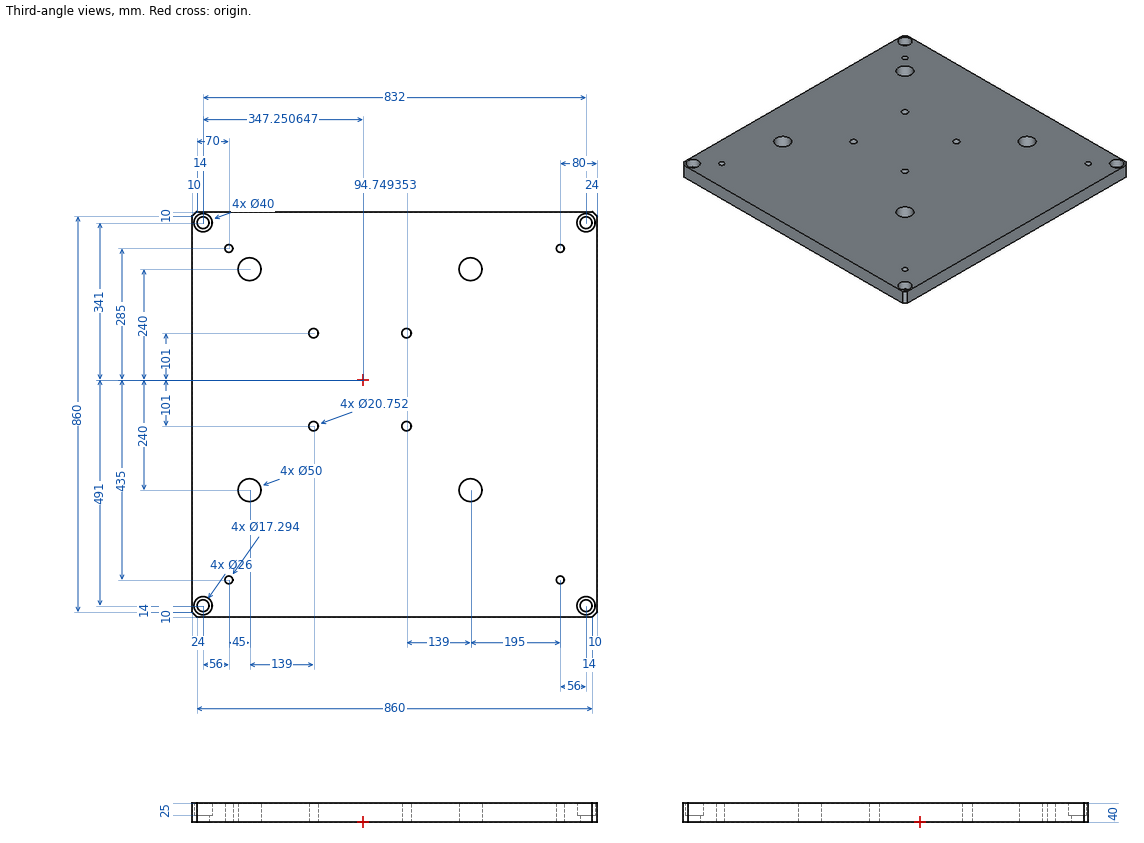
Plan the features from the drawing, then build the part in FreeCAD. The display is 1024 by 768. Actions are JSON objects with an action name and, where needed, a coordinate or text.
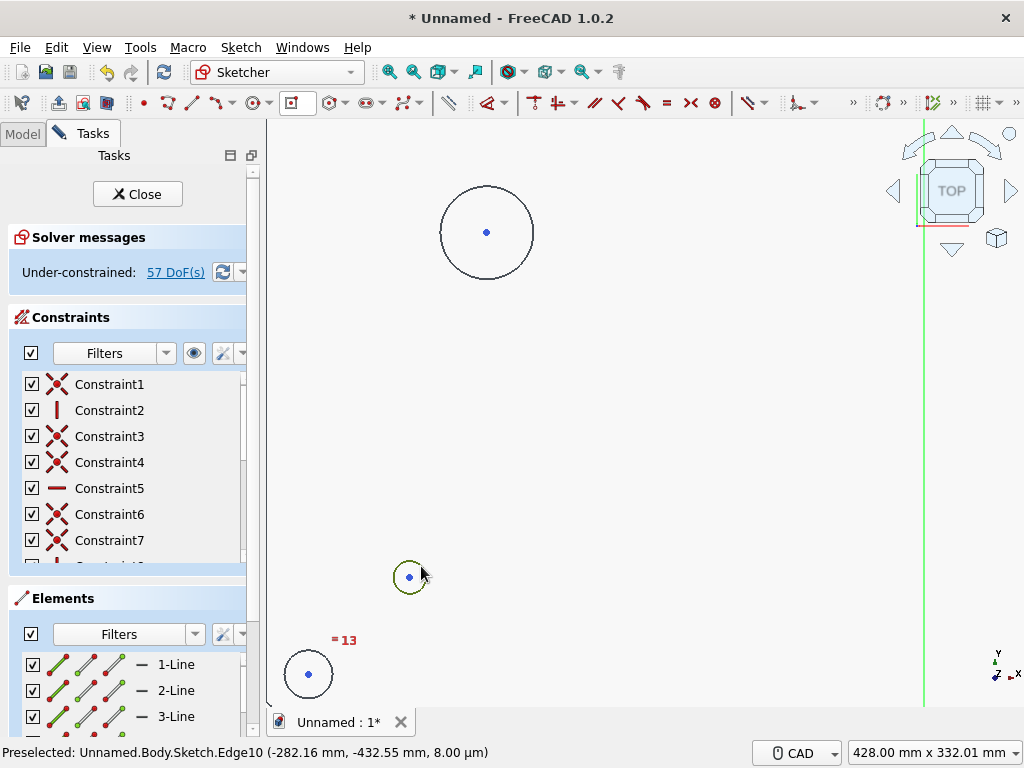
{"action": "scroll", "coordinate": [423, 569], "scroll_direction": "down", "scroll_amount": 7}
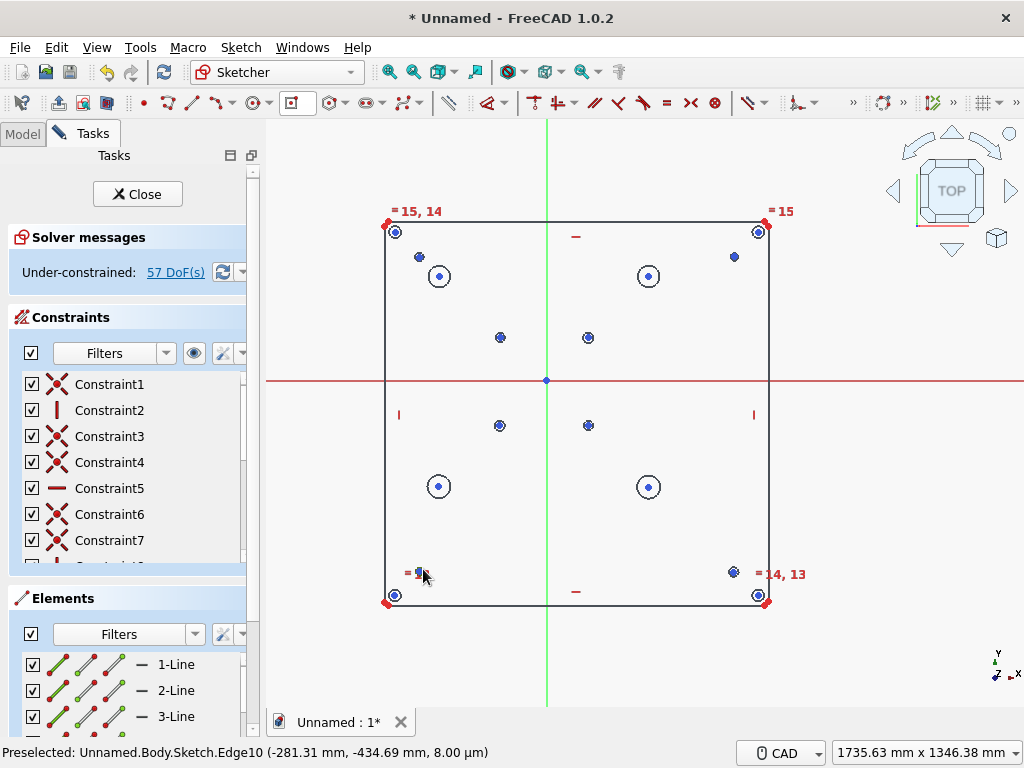
{"action": "scroll", "coordinate": [737, 569], "scroll_direction": "up", "scroll_amount": 6}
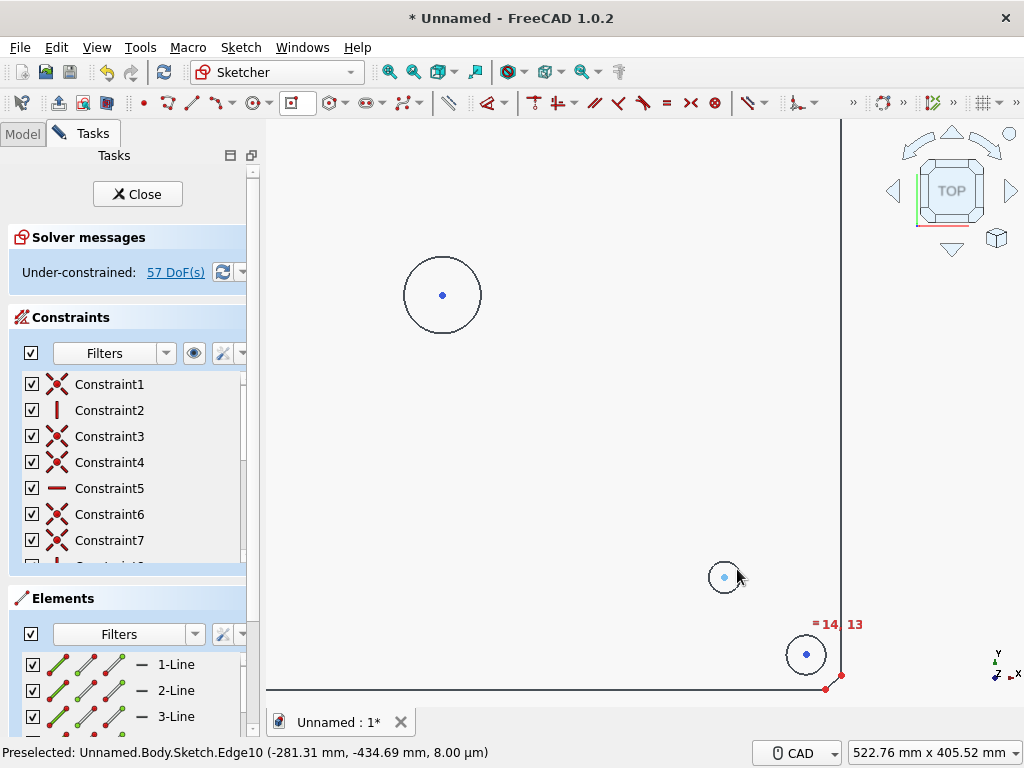
{"action": "left_click", "coordinate": [736, 566]}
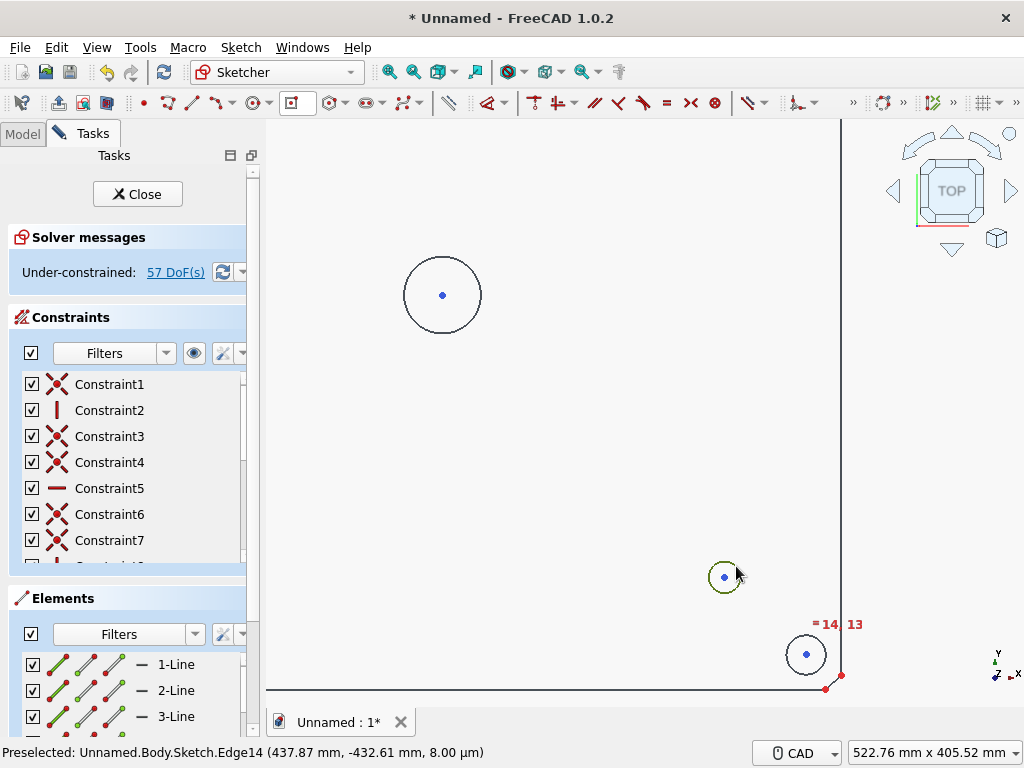
{"action": "scroll", "coordinate": [737, 569], "scroll_direction": "down", "scroll_amount": 6}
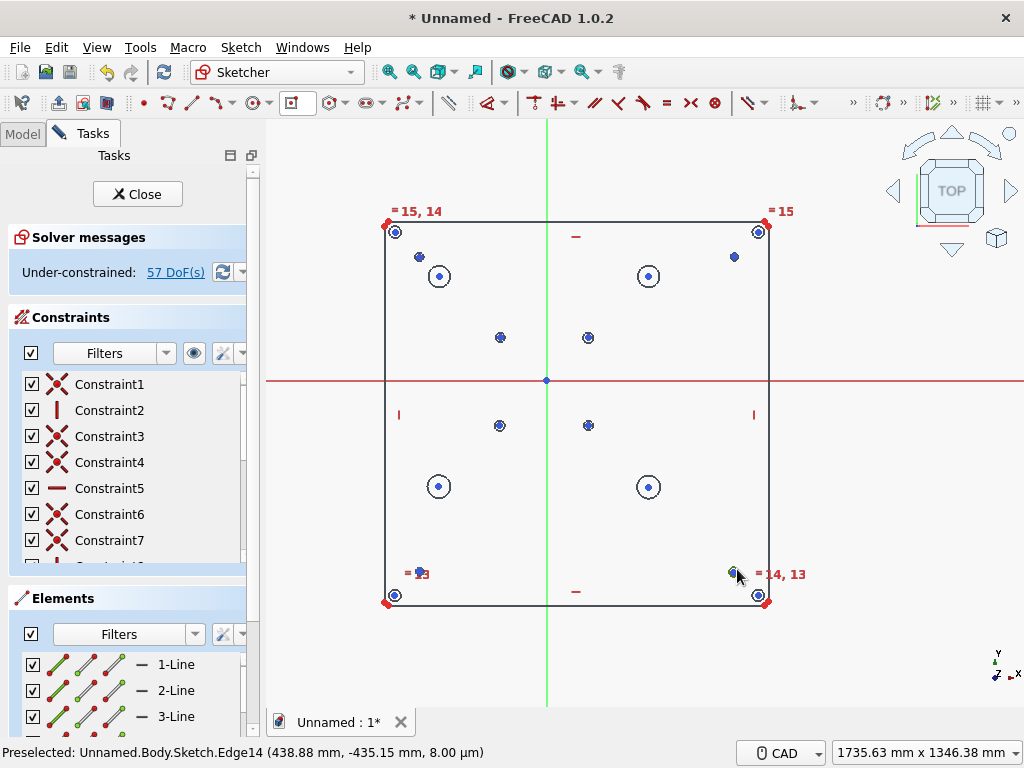
{"action": "scroll", "coordinate": [422, 254], "scroll_direction": "up", "scroll_amount": 6}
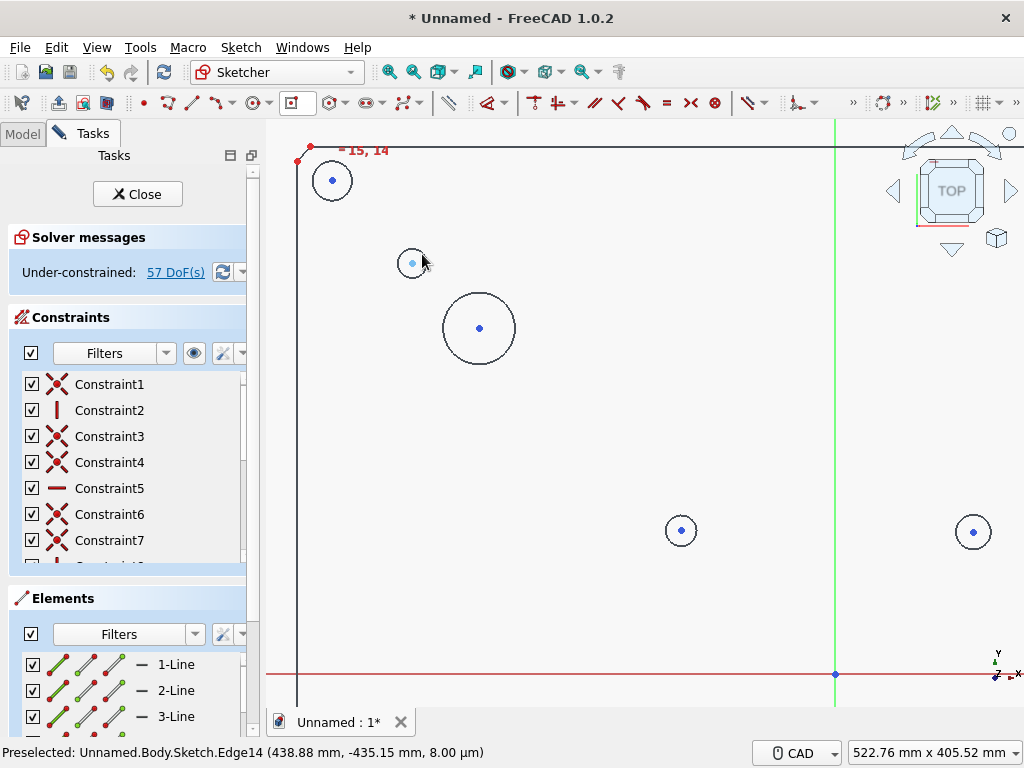
{"action": "left_click", "coordinate": [423, 253]}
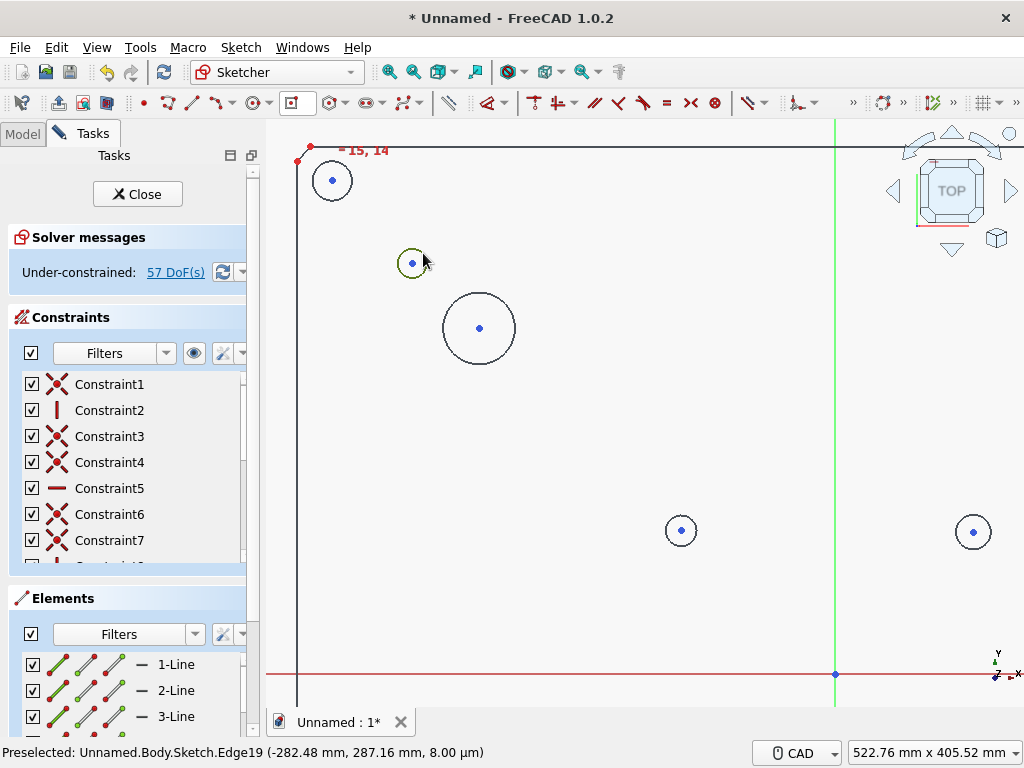
{"action": "scroll", "coordinate": [422, 253], "scroll_direction": "down", "scroll_amount": 6}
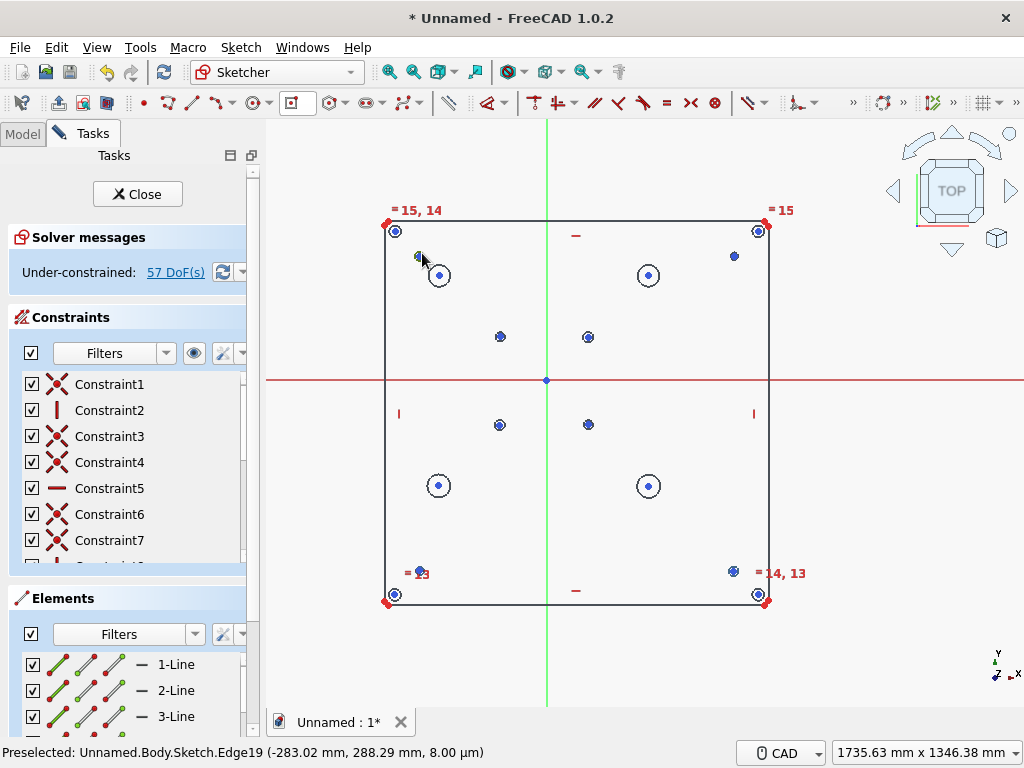
{"action": "scroll", "coordinate": [737, 254], "scroll_direction": "up", "scroll_amount": 7}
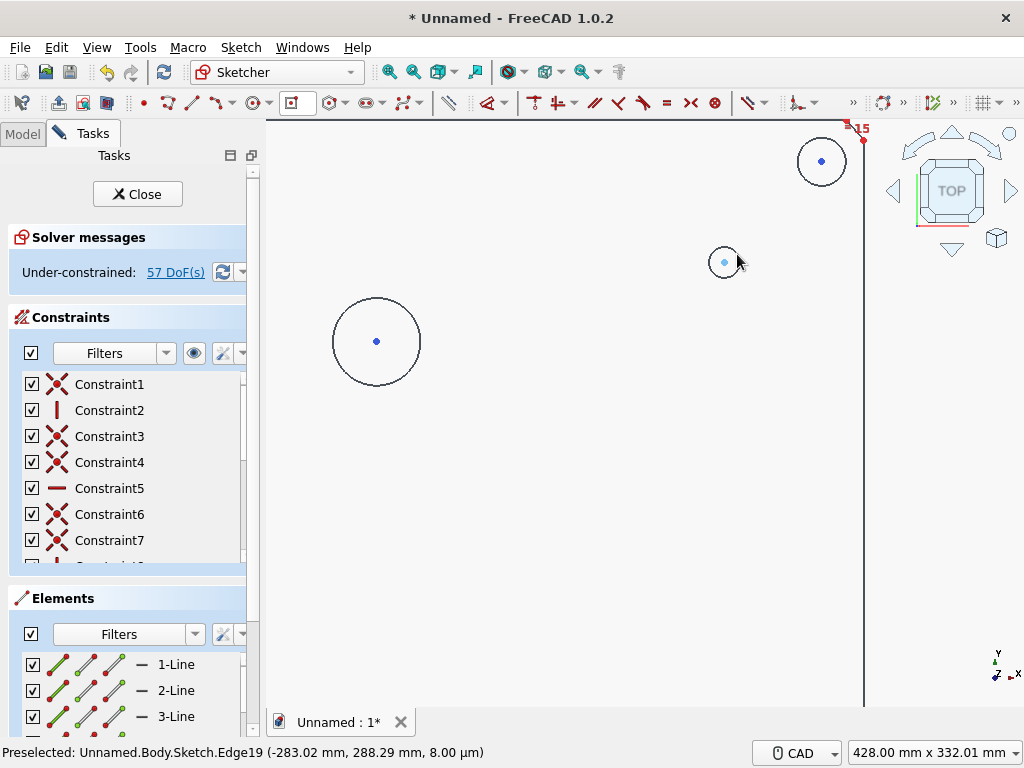
{"action": "left_click", "coordinate": [735, 252]}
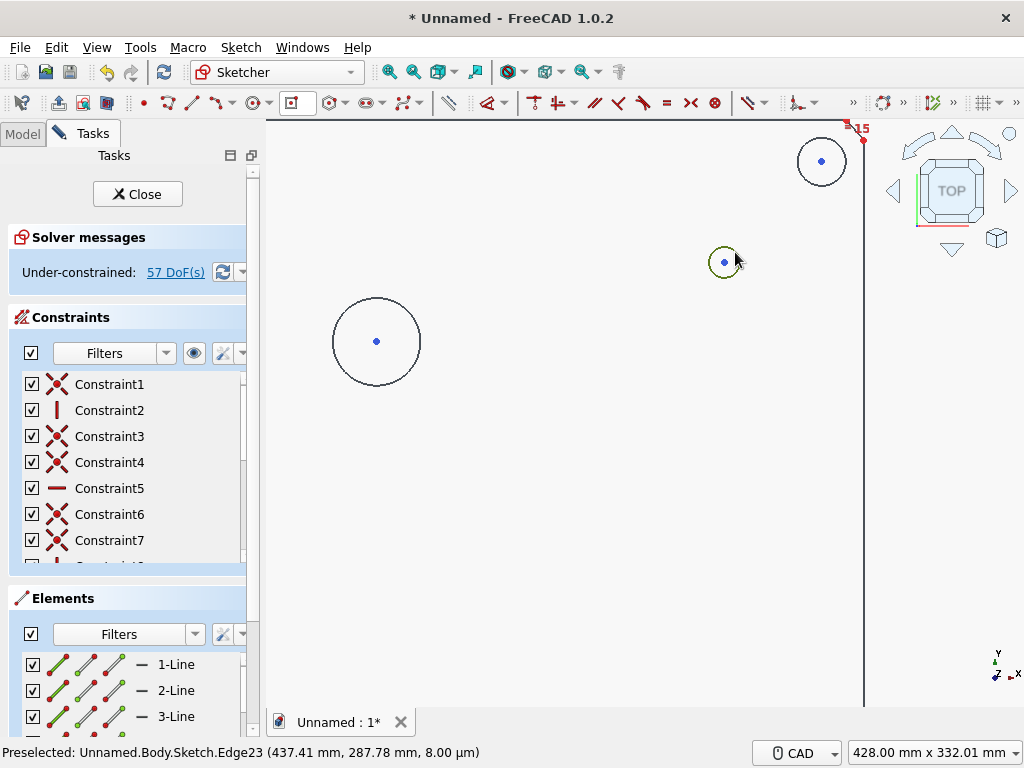
{"action": "key", "text": "e"}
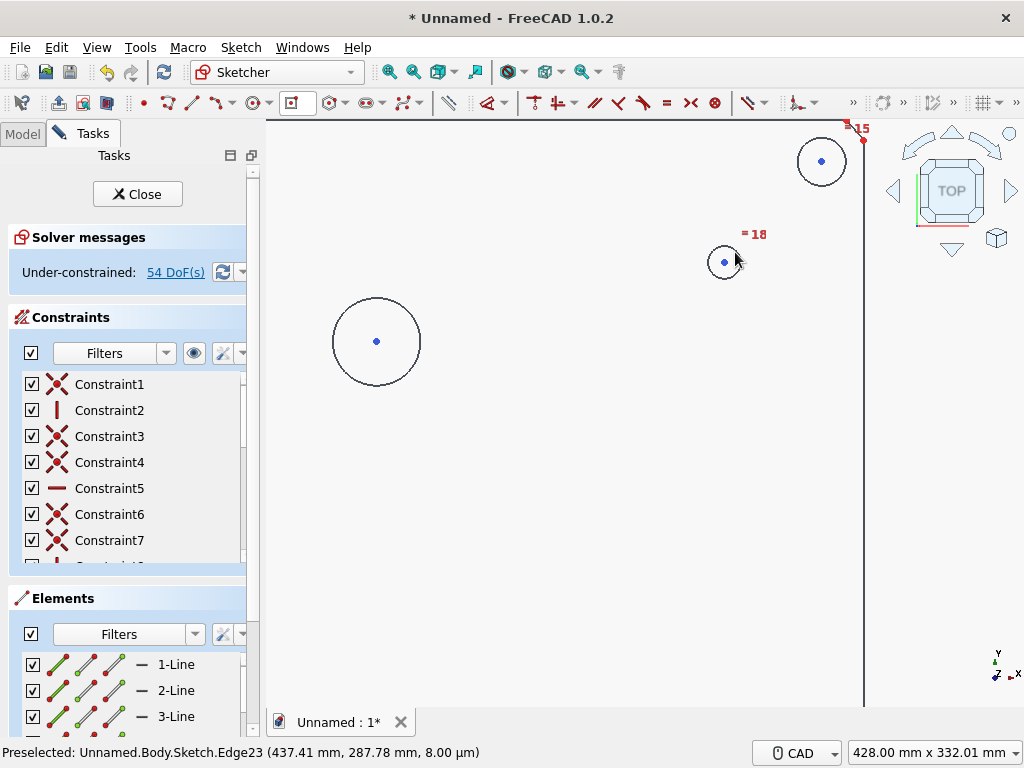
{"action": "scroll", "coordinate": [737, 254], "scroll_direction": "down", "scroll_amount": 7}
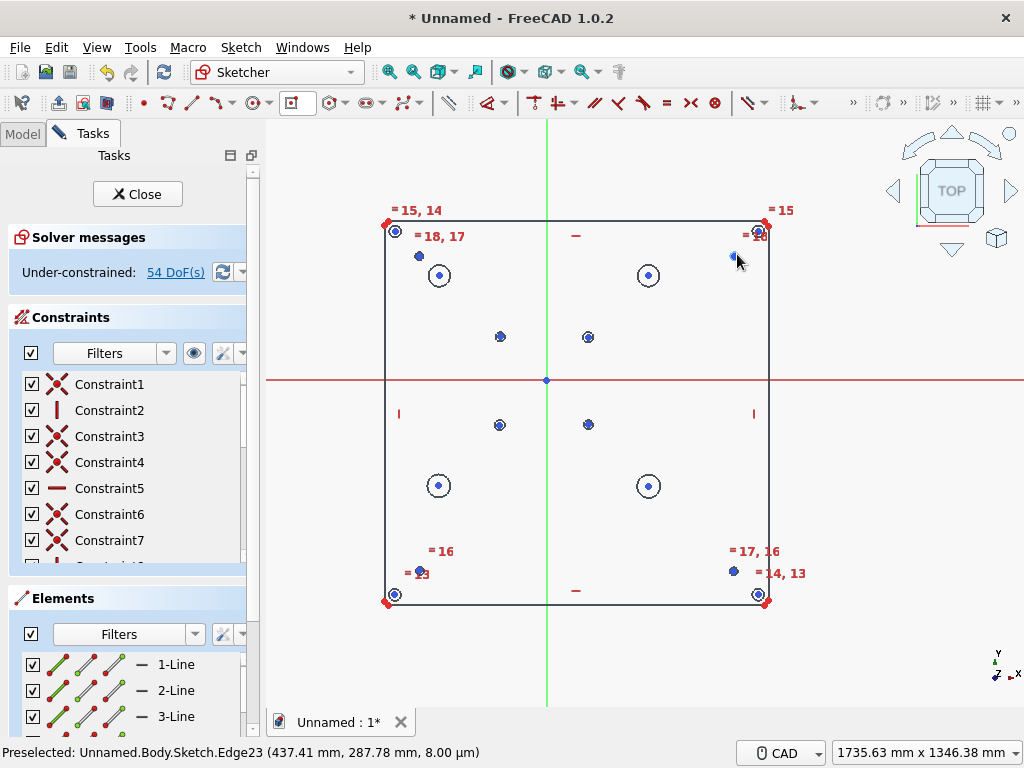
{"action": "left_click", "coordinate": [447, 478]}